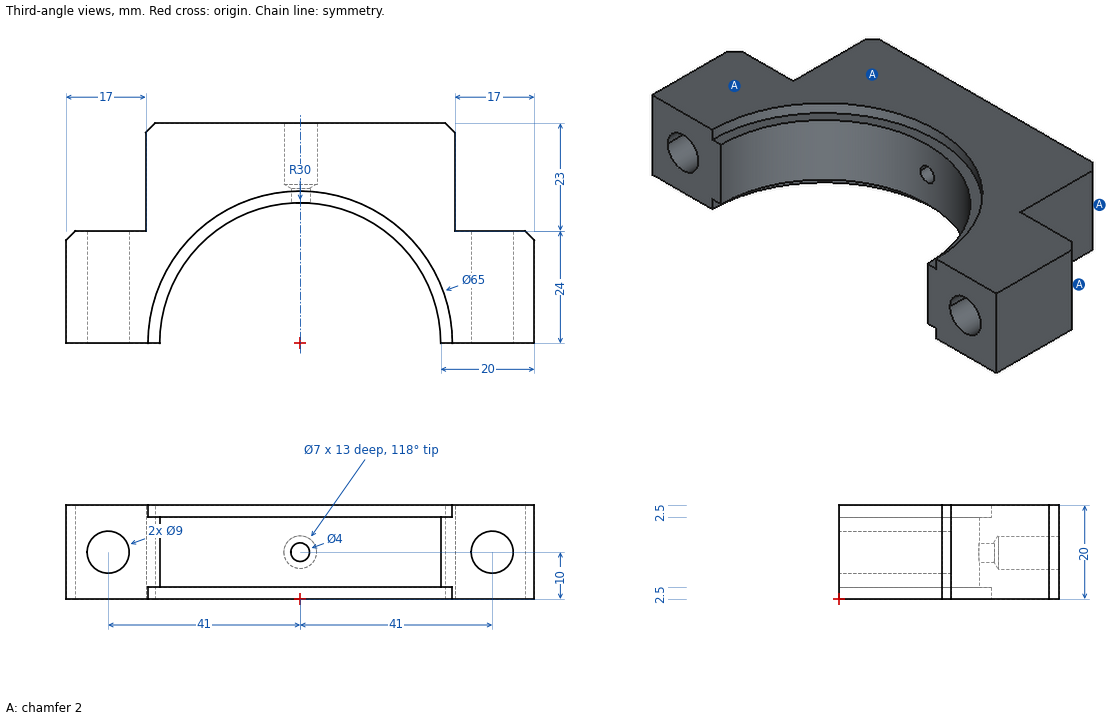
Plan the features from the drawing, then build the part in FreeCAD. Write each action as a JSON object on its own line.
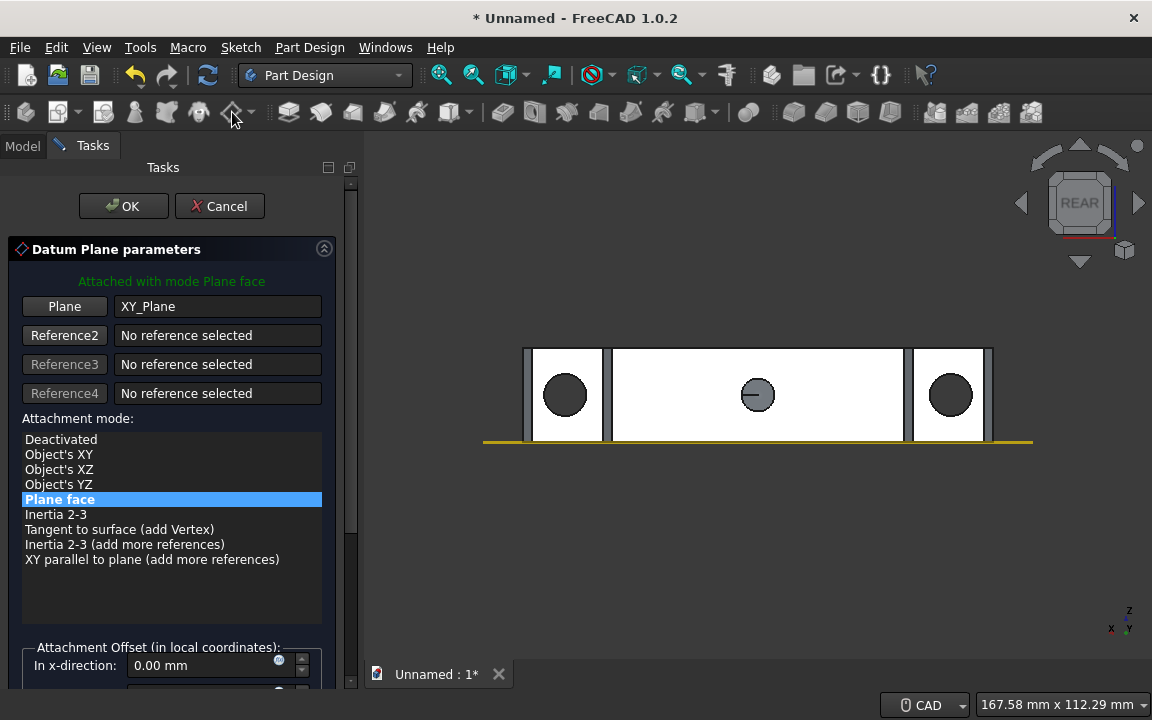
{"action": "scroll", "coordinate": [351, 432], "scroll_direction": "down", "scroll_amount": 2}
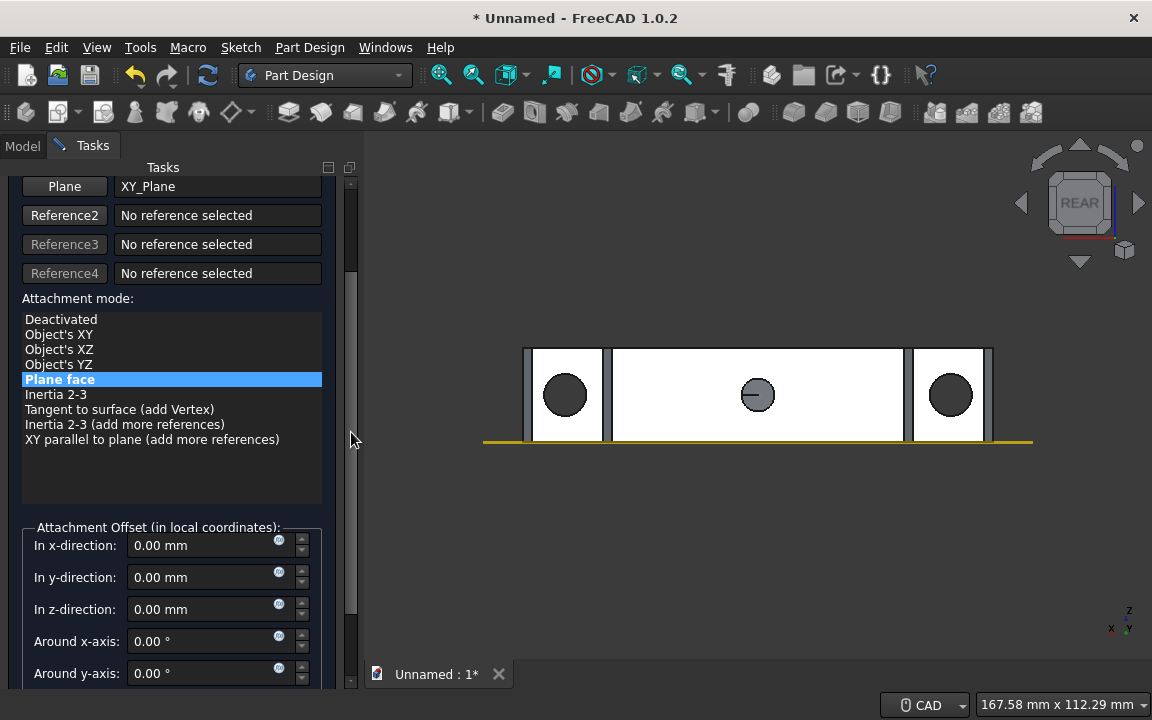
{"action": "triple_click", "coordinate": [210, 609]}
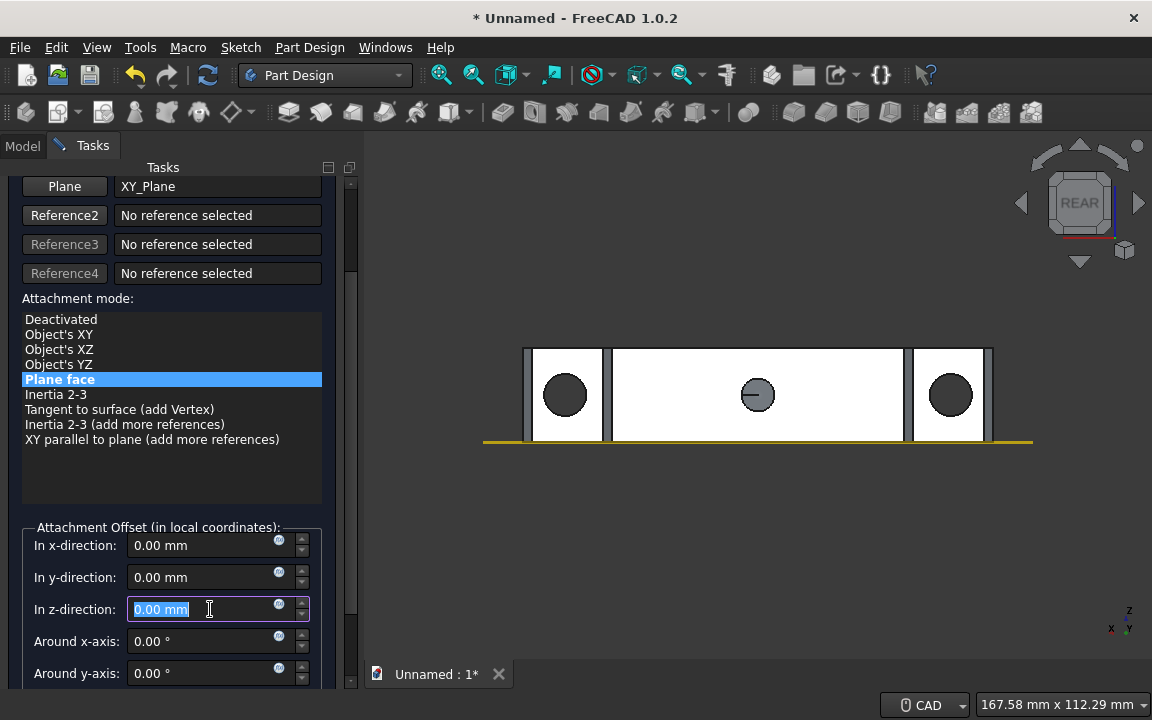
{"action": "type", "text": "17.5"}
{"action": "key", "text": "Tab"}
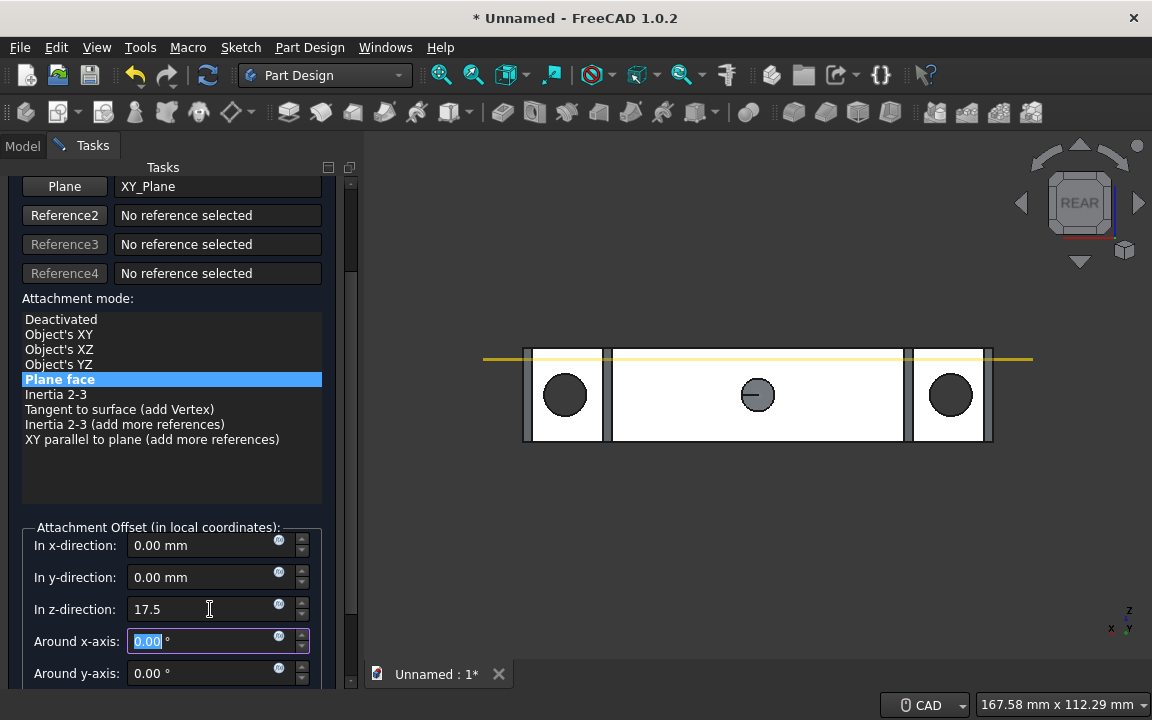
{"action": "scroll", "coordinate": [351, 432], "scroll_direction": "up", "scroll_amount": 3}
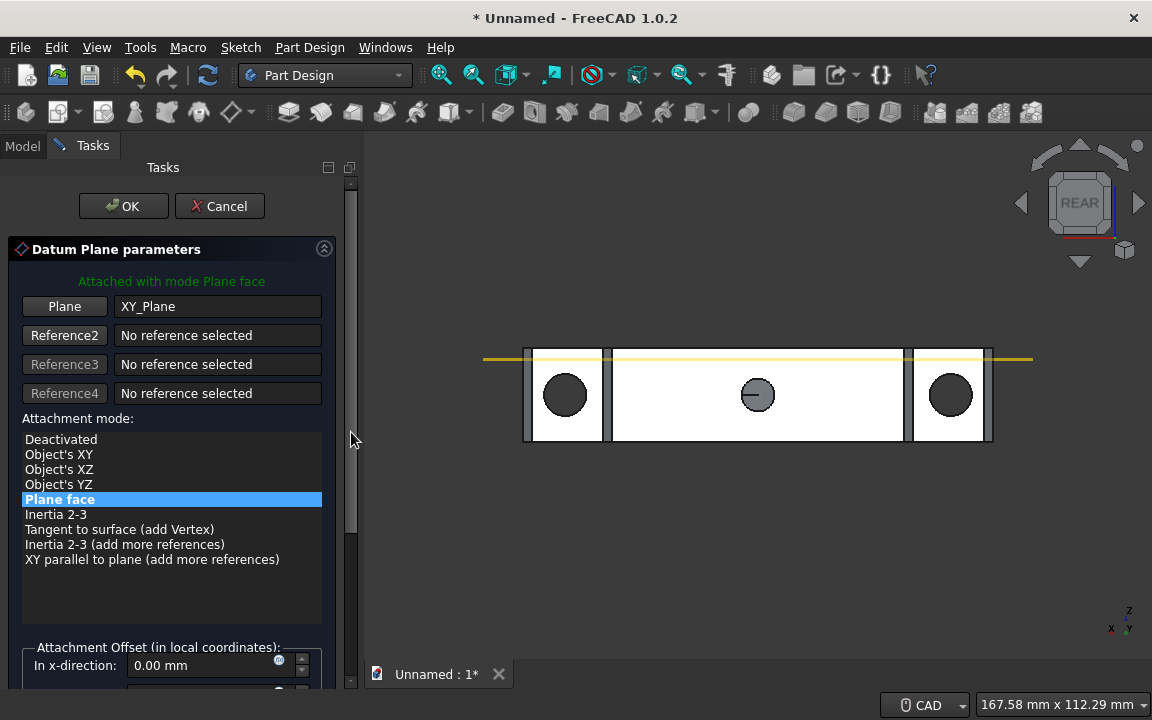
{"action": "left_click", "coordinate": [124, 206]}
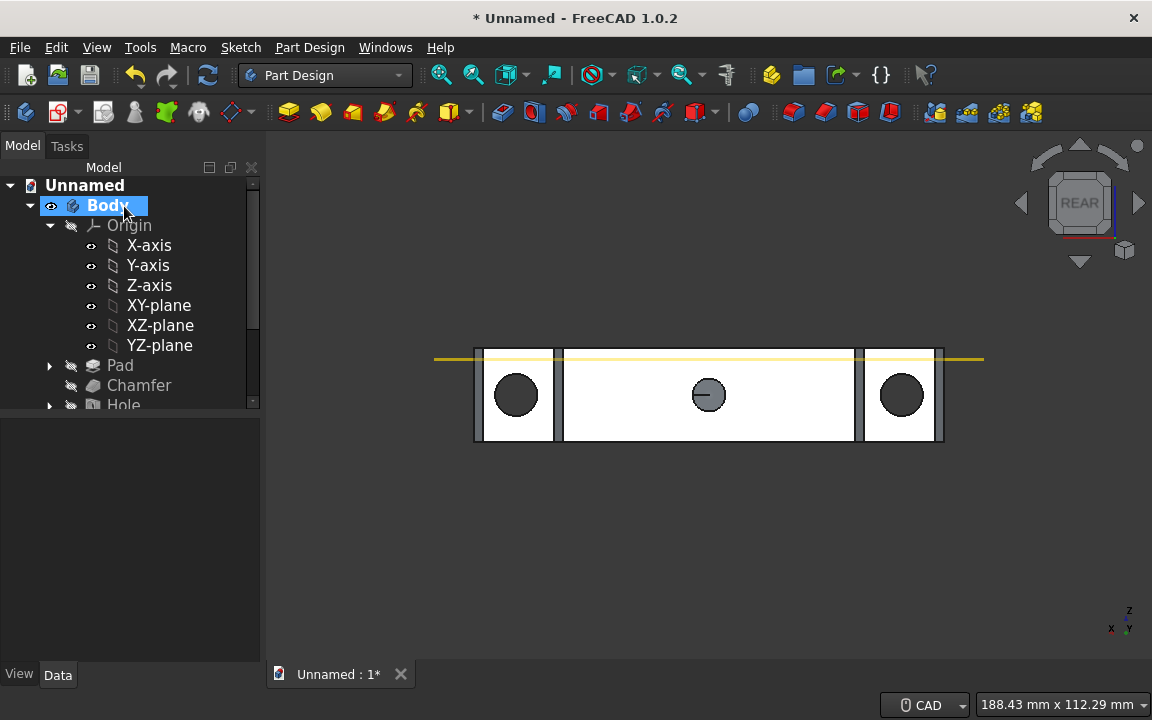
{"action": "scroll", "coordinate": [100, 301], "scroll_direction": "down", "scroll_amount": 3}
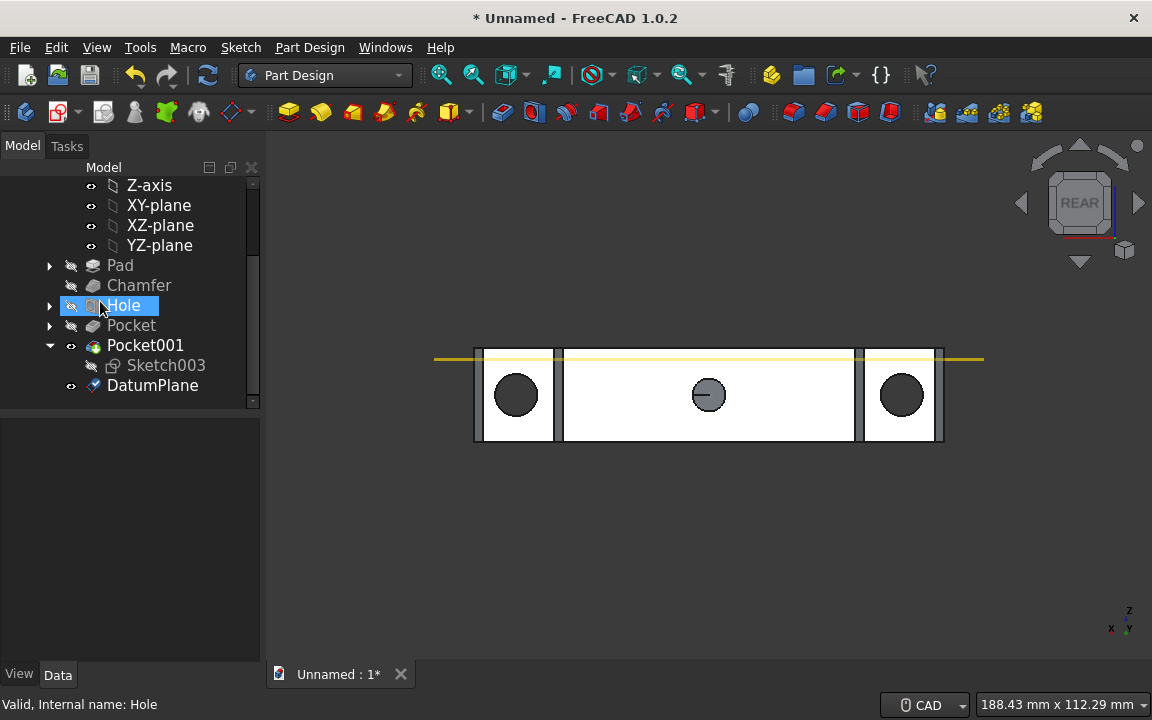
{"action": "left_click", "coordinate": [116, 386]}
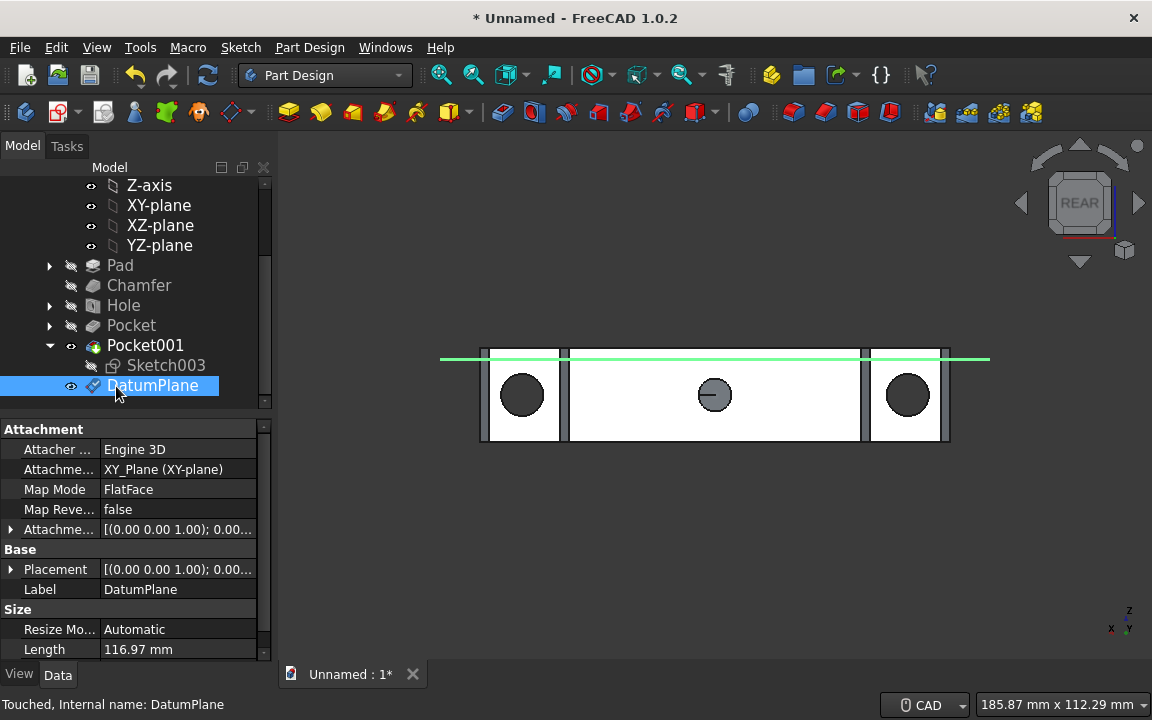
{"action": "left_click", "coordinate": [58, 112]}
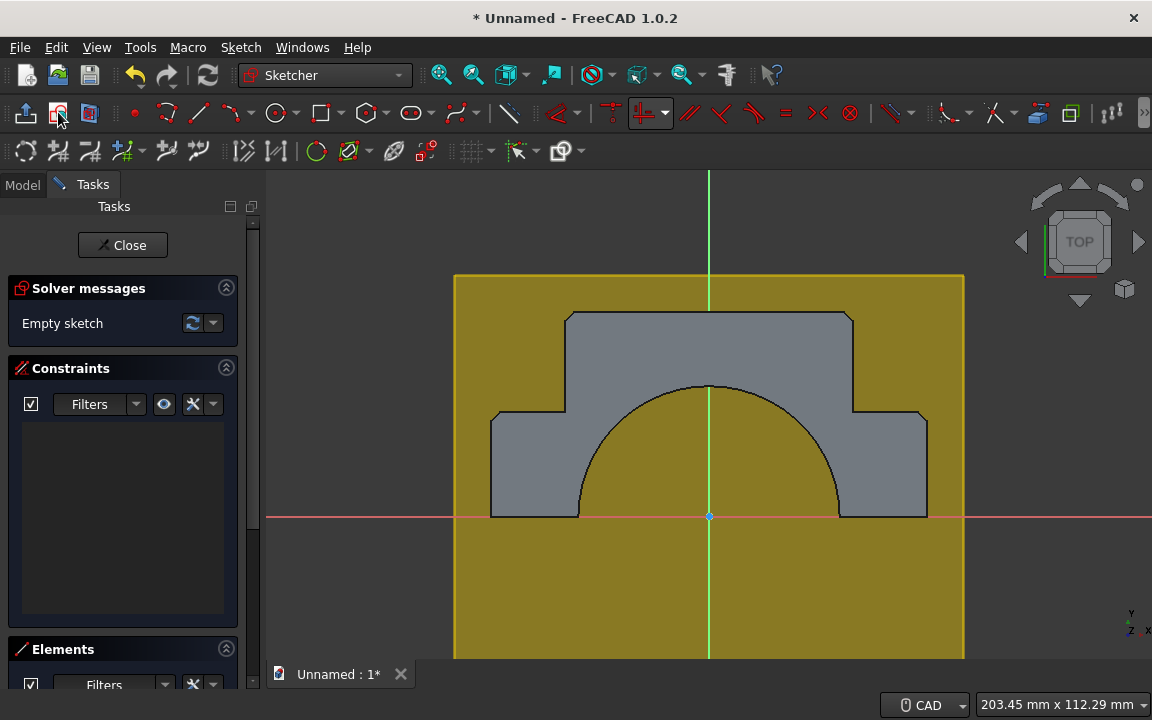
{"action": "left_click", "coordinate": [90, 114]}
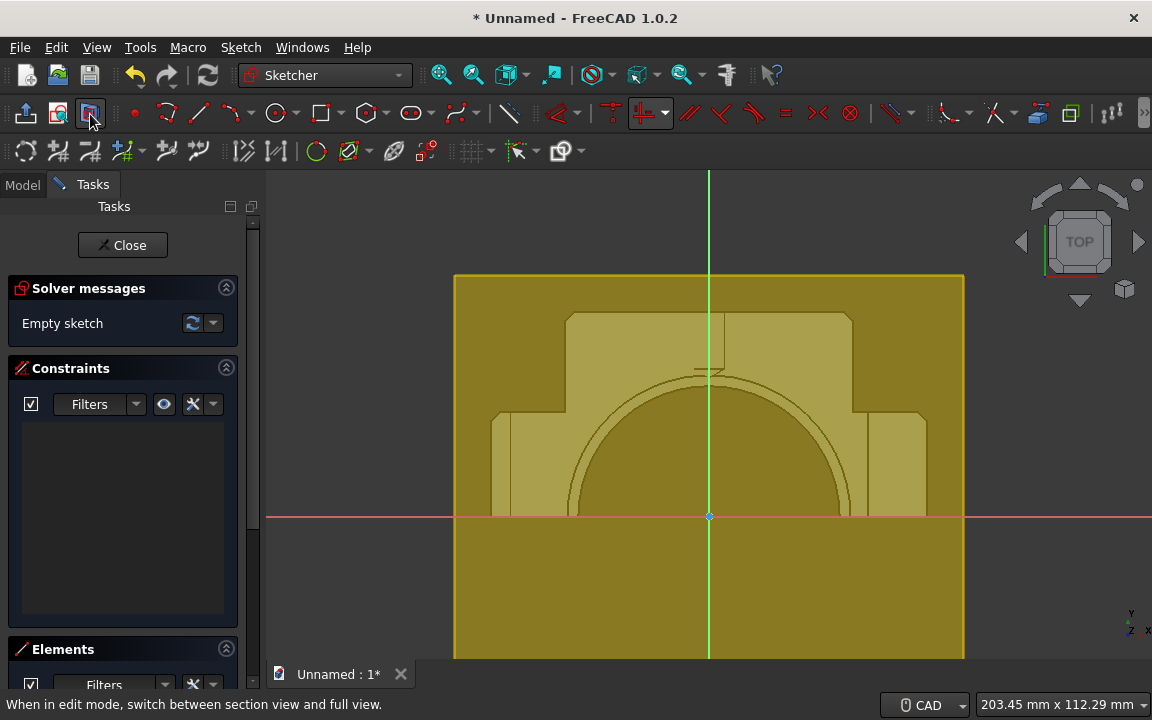
{"action": "scroll", "coordinate": [331, 198], "scroll_direction": "down", "scroll_amount": 1}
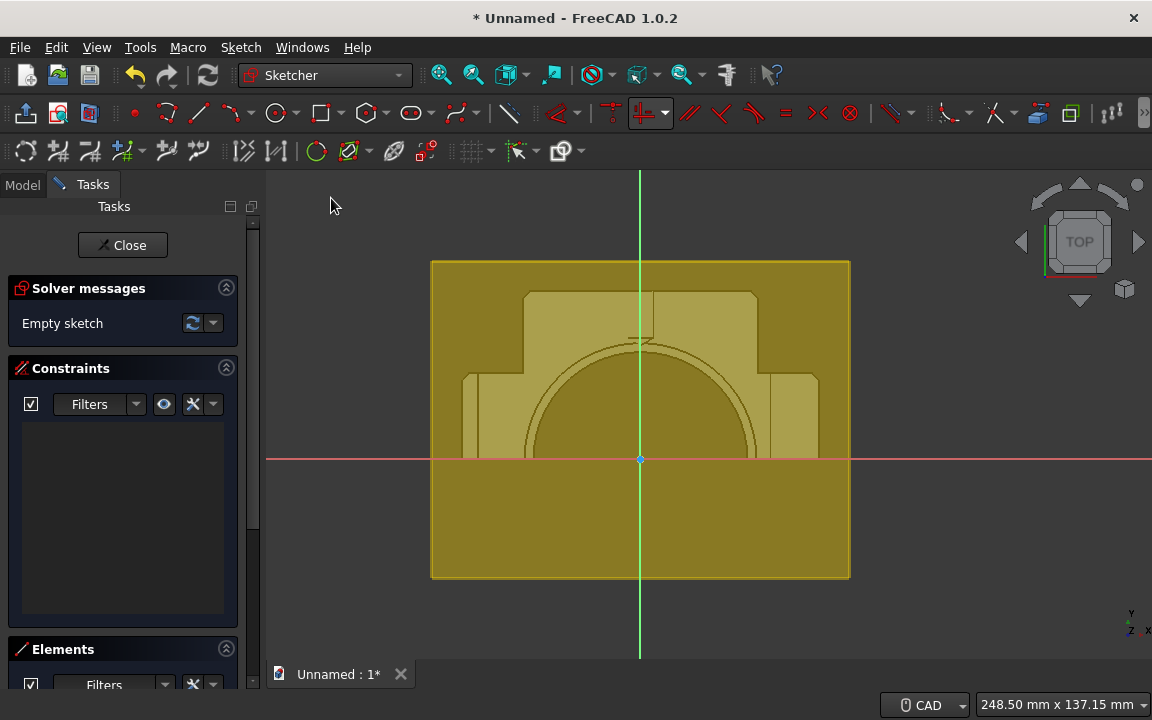
{"action": "left_click", "coordinate": [276, 114]}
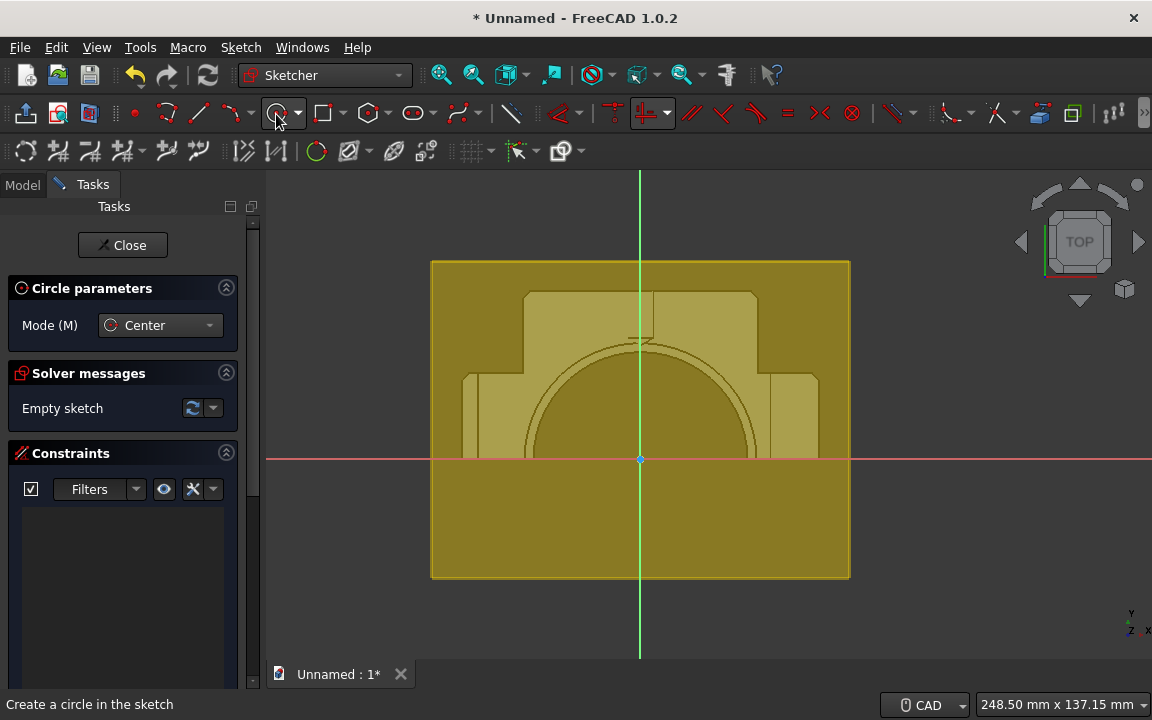
{"action": "left_click", "coordinate": [640, 459]}
{"action": "mouse_move", "coordinate": [722, 377]}